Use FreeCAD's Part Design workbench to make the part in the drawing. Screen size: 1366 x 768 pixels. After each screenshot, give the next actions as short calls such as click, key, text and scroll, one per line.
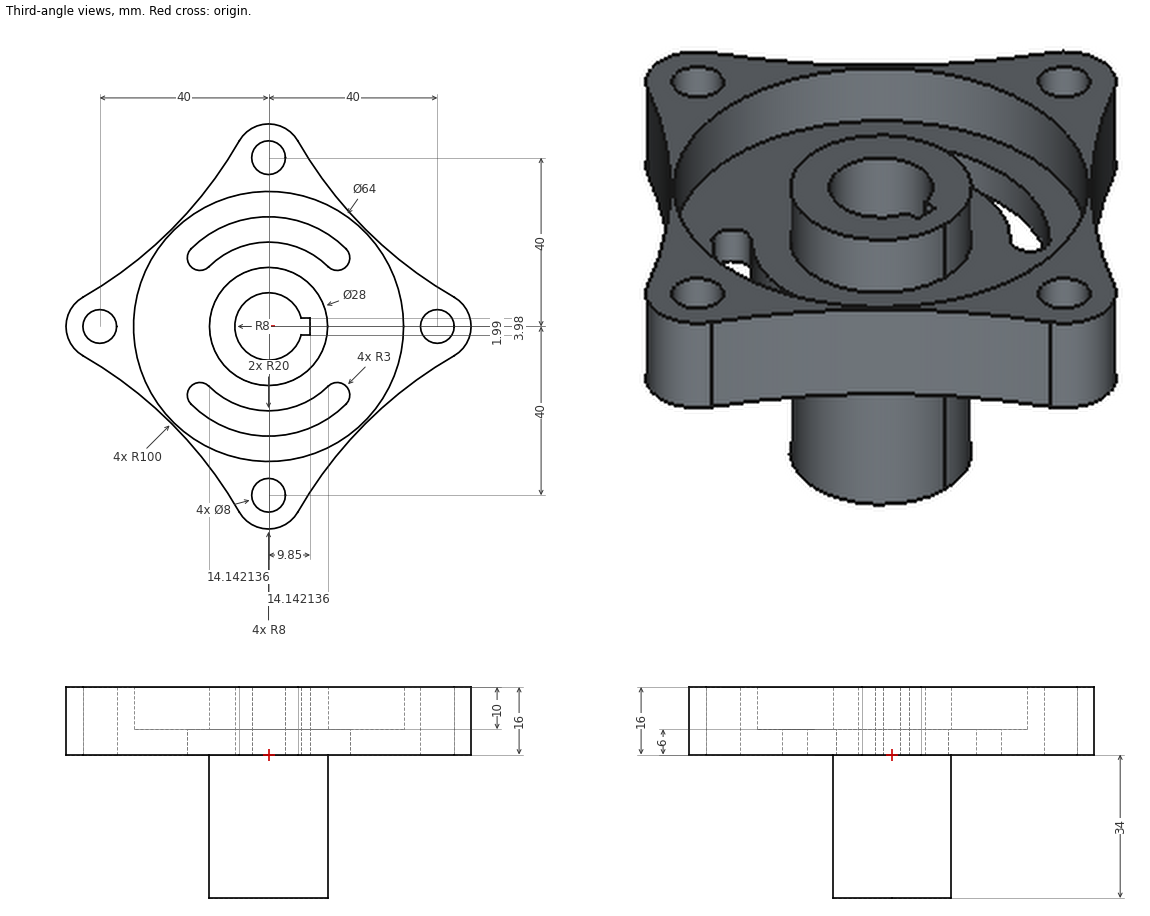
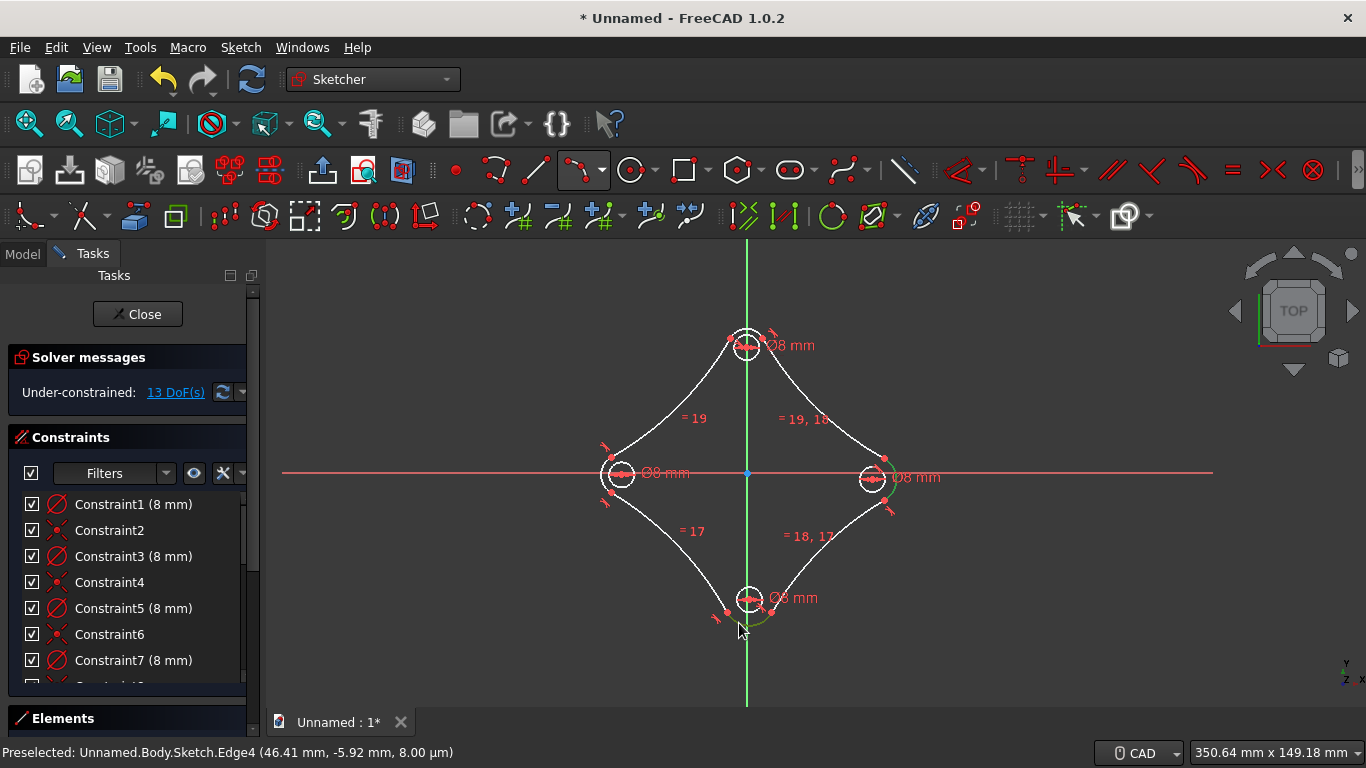
scroll(754, 330, up, 5)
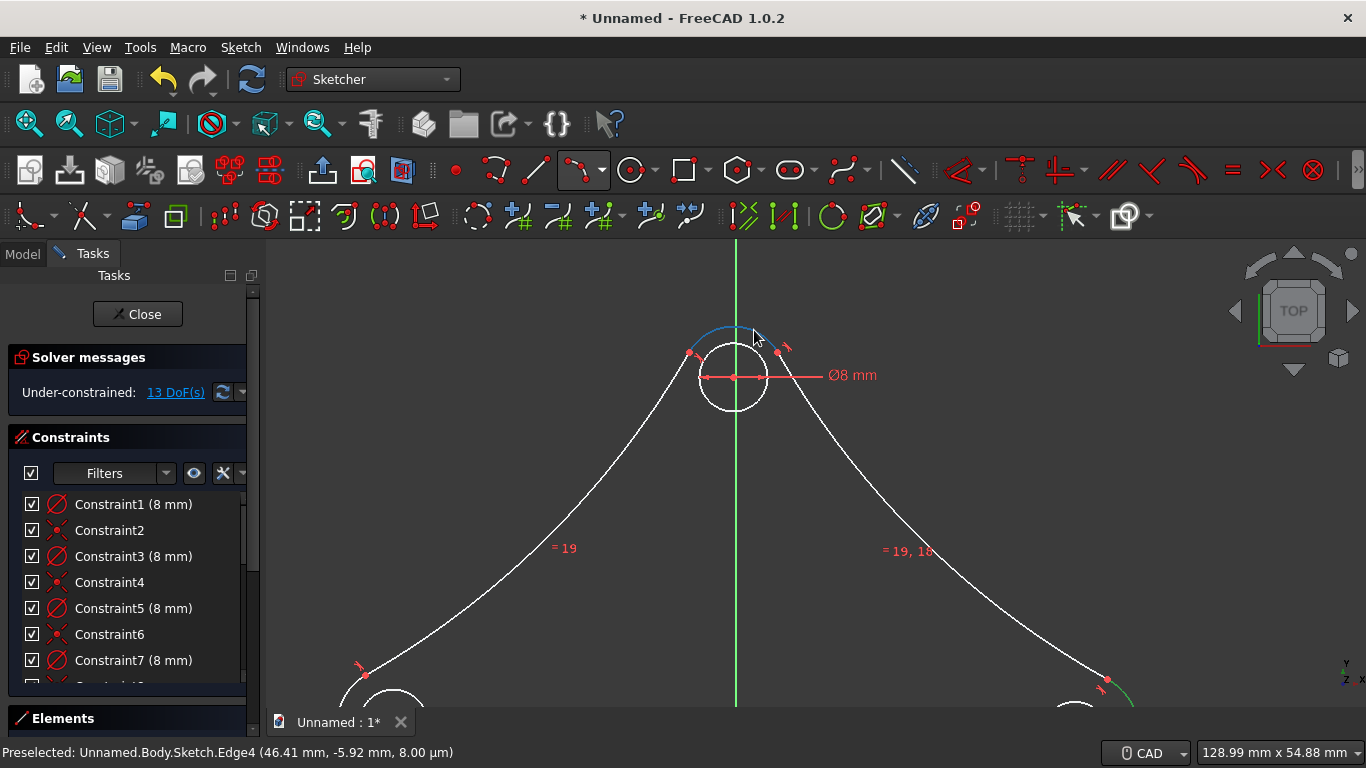
click(754, 331)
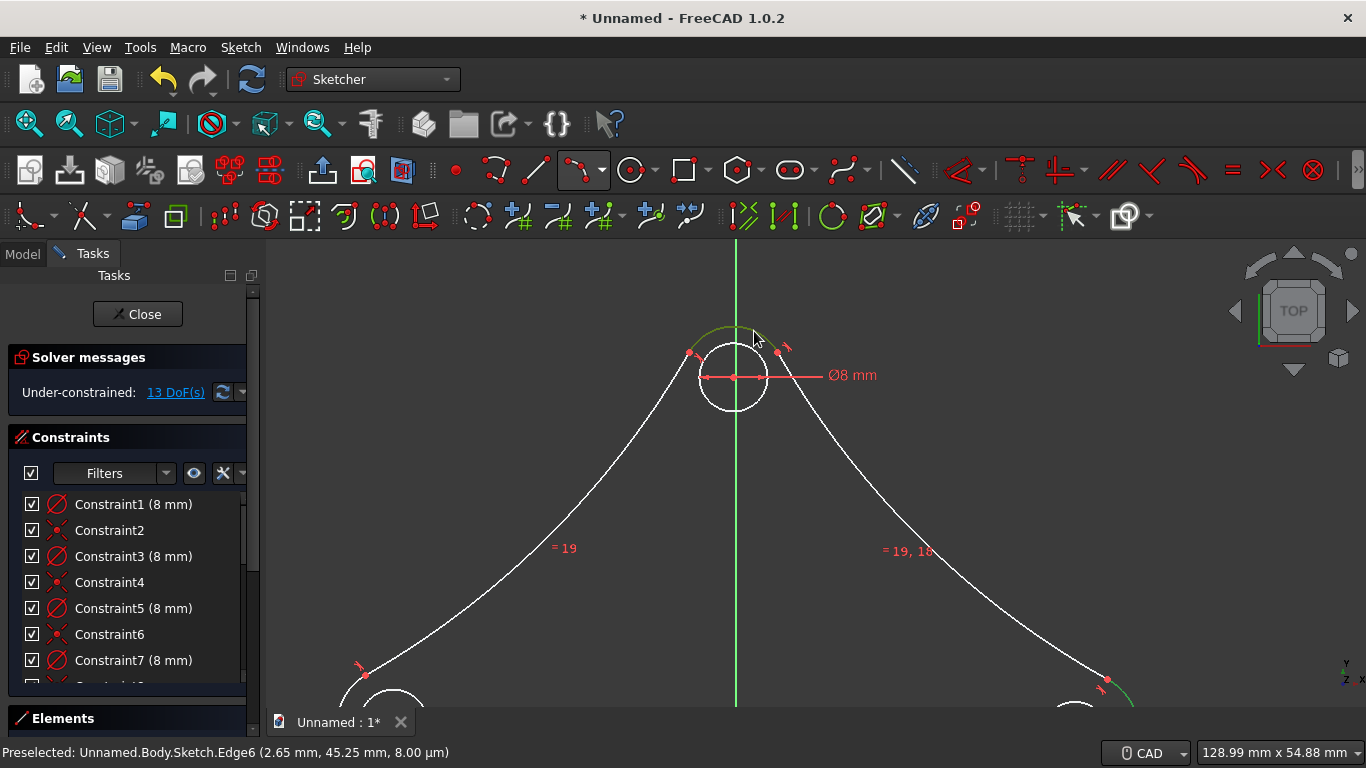
scroll(754, 330, down, 5)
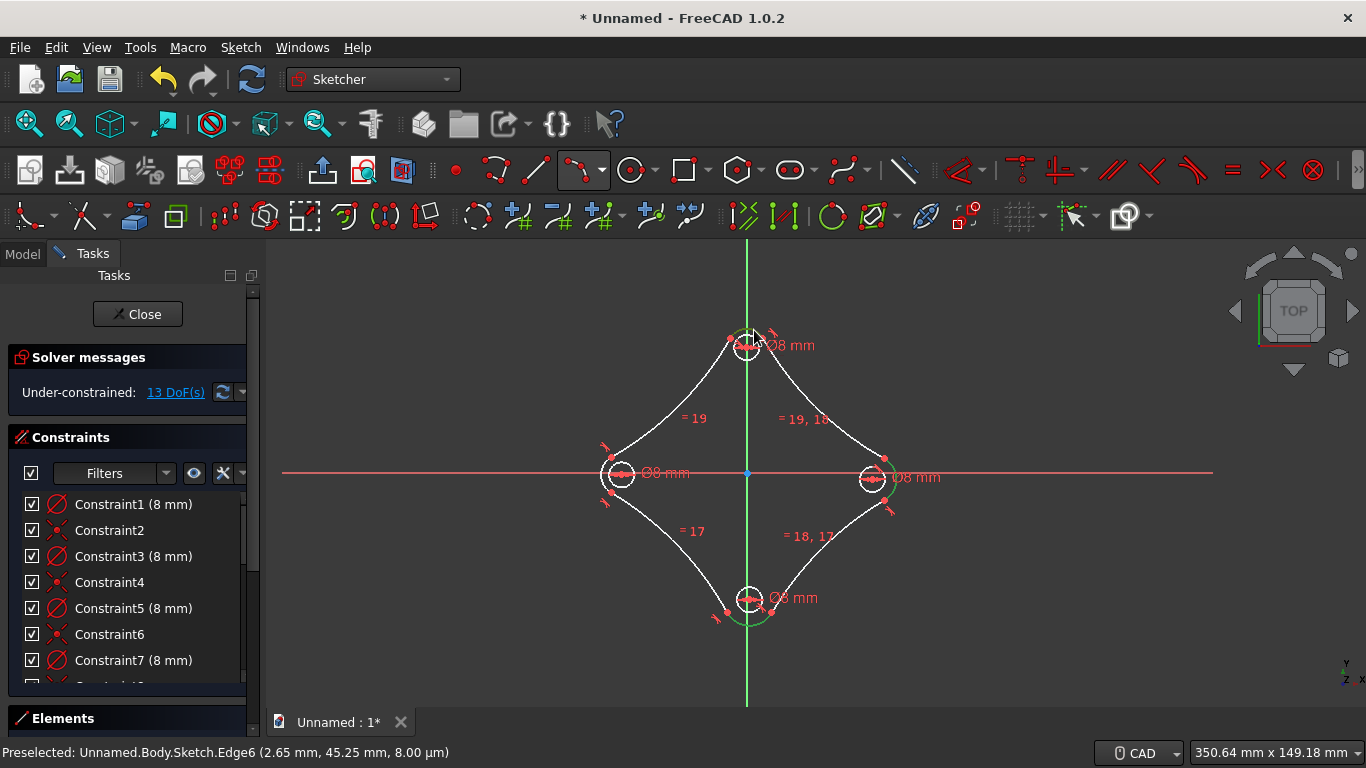
scroll(603, 466, up, 4)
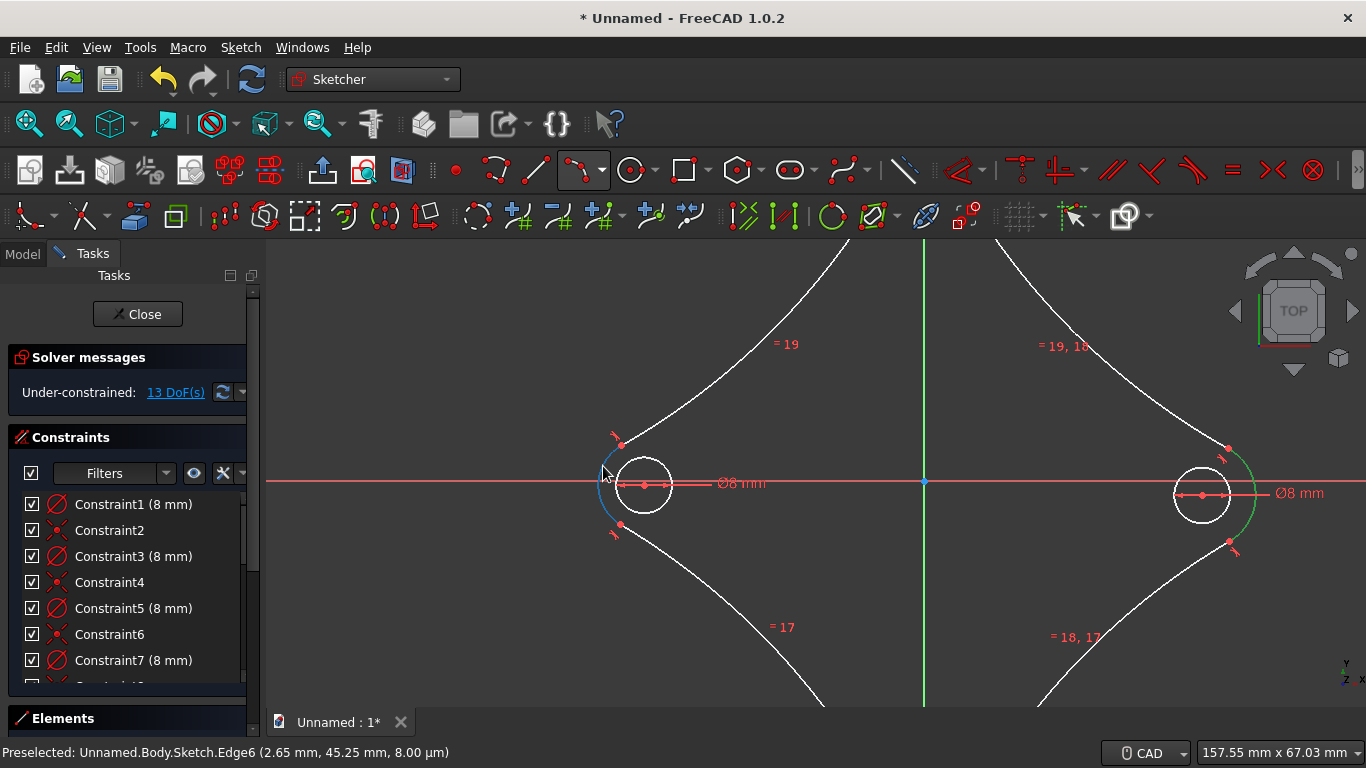
click(602, 466)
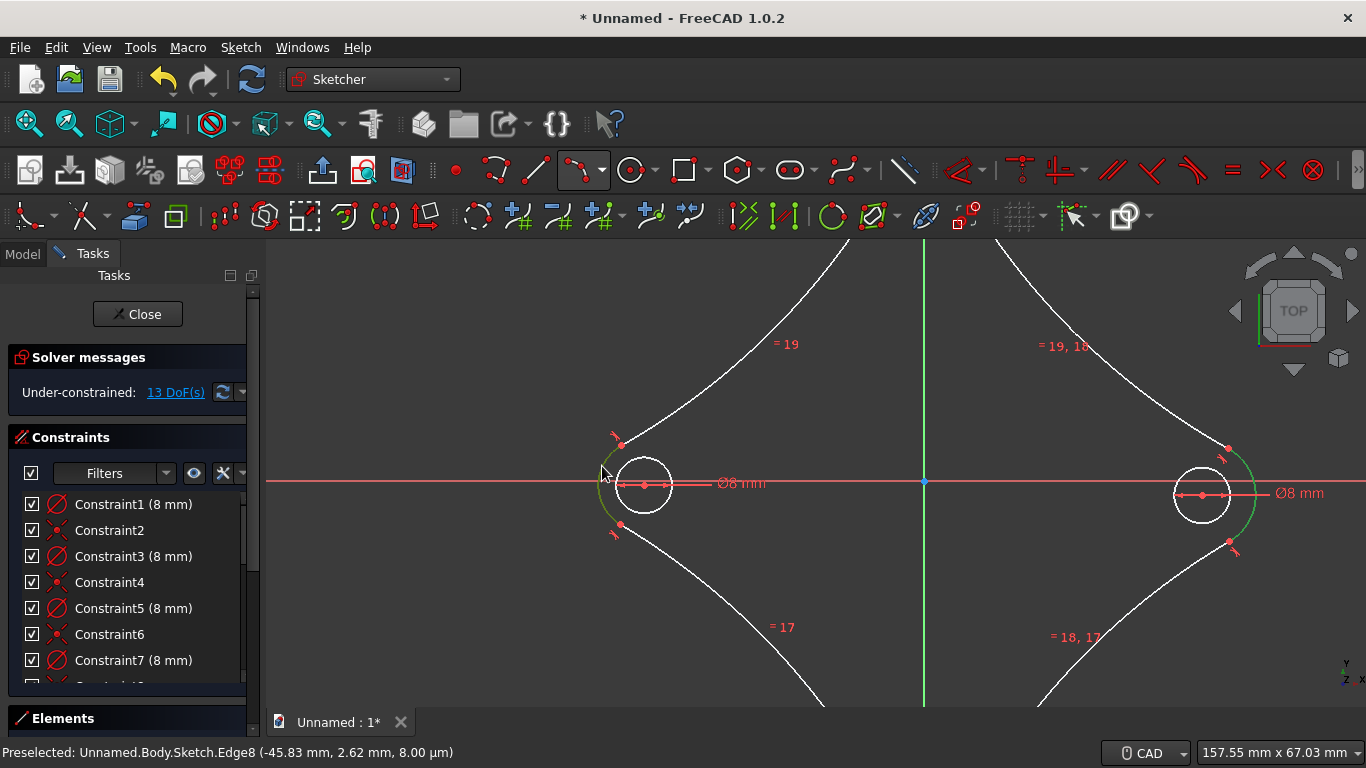
click(1234, 170)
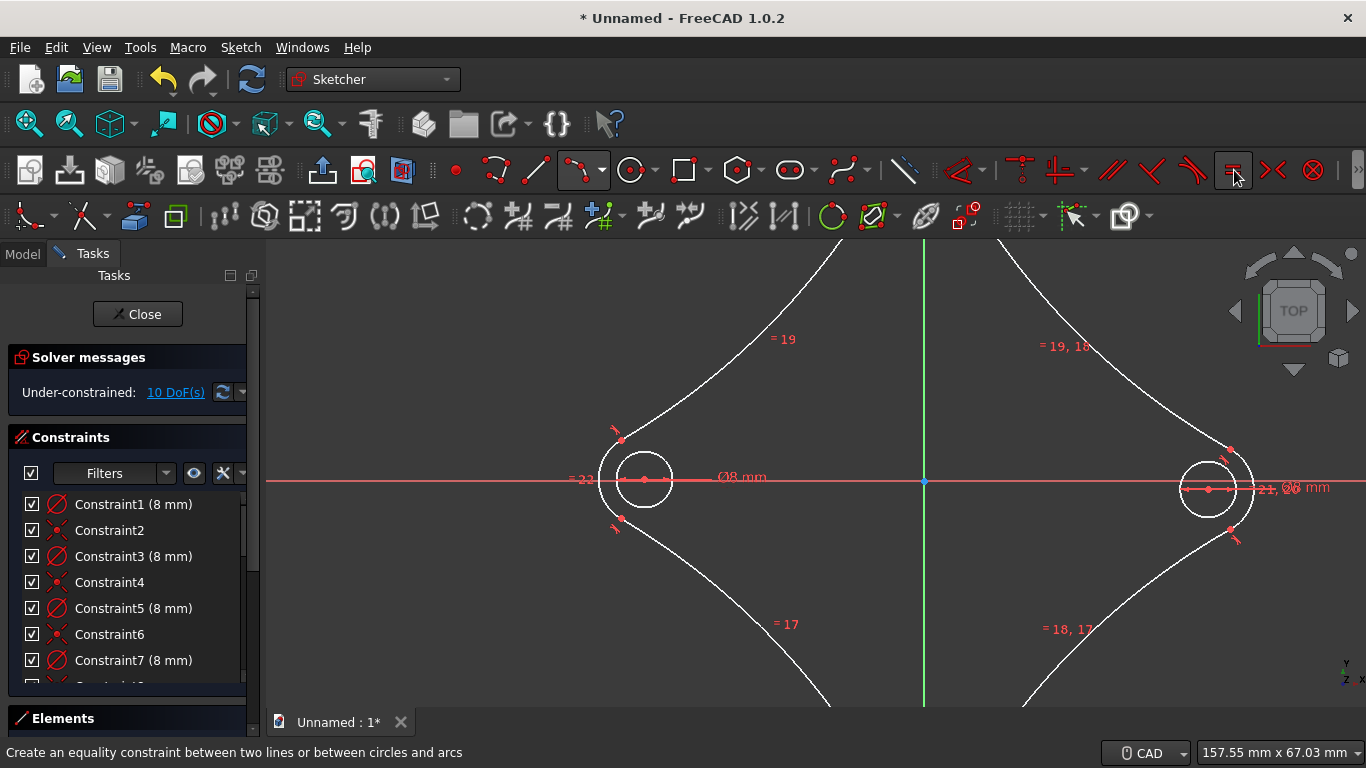
scroll(603, 466, down, 4)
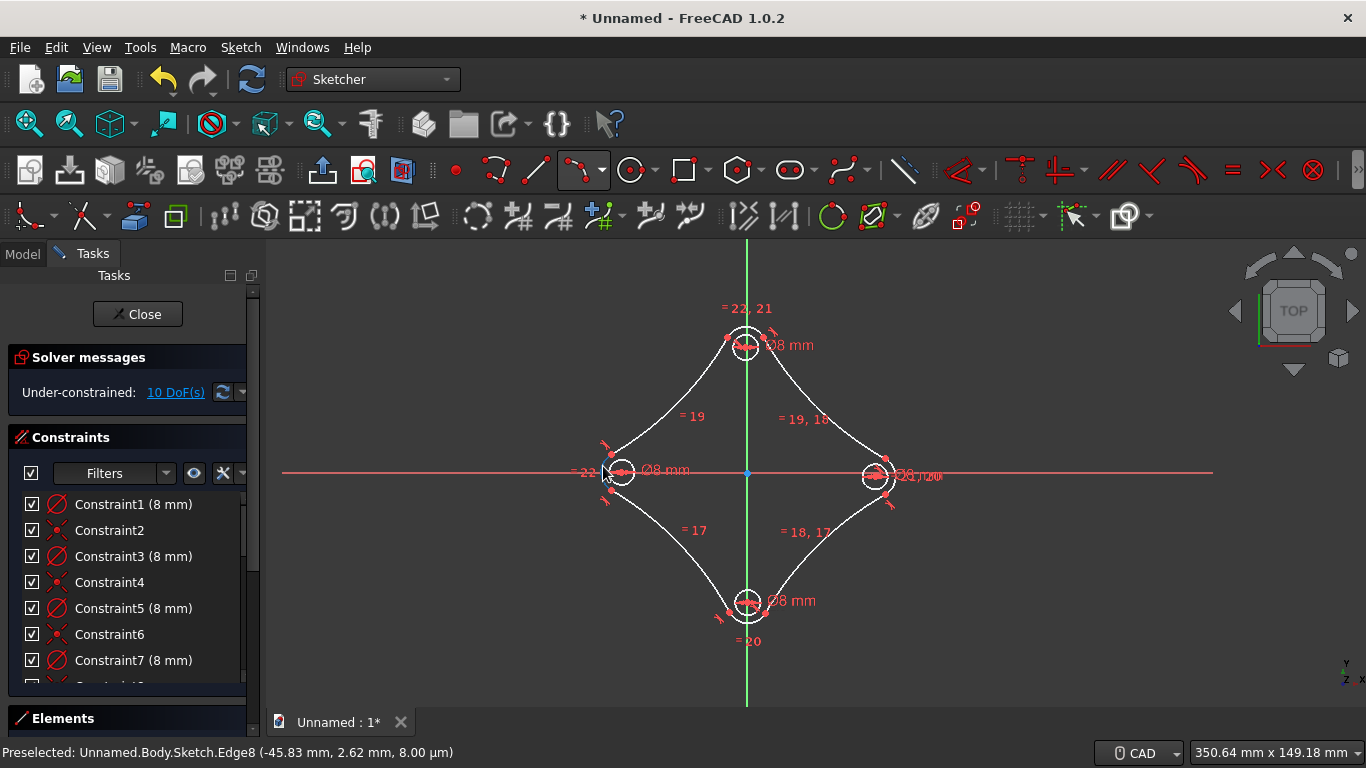
click(748, 603)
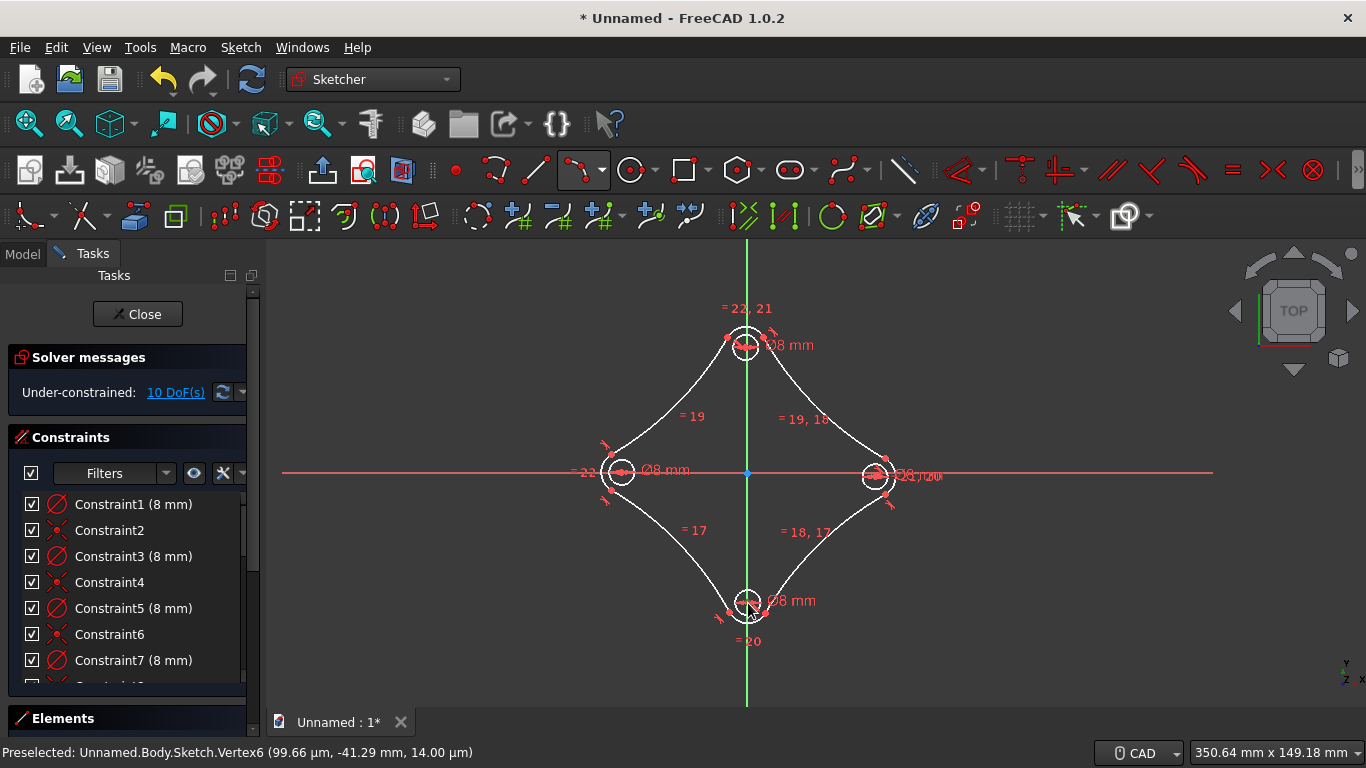
click(747, 532)